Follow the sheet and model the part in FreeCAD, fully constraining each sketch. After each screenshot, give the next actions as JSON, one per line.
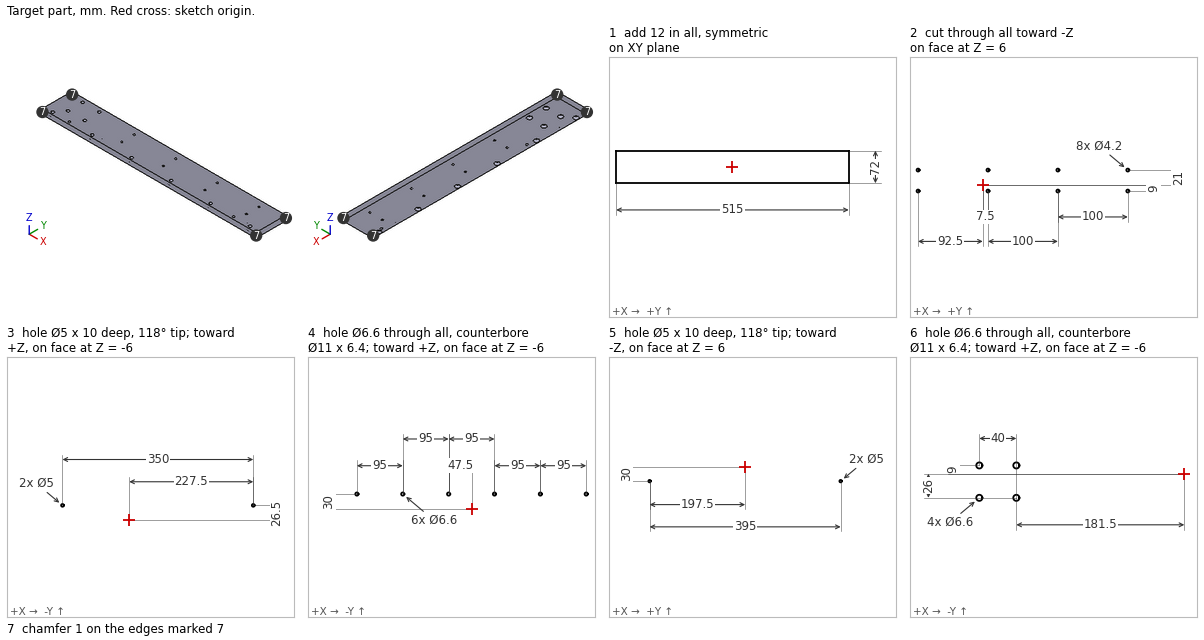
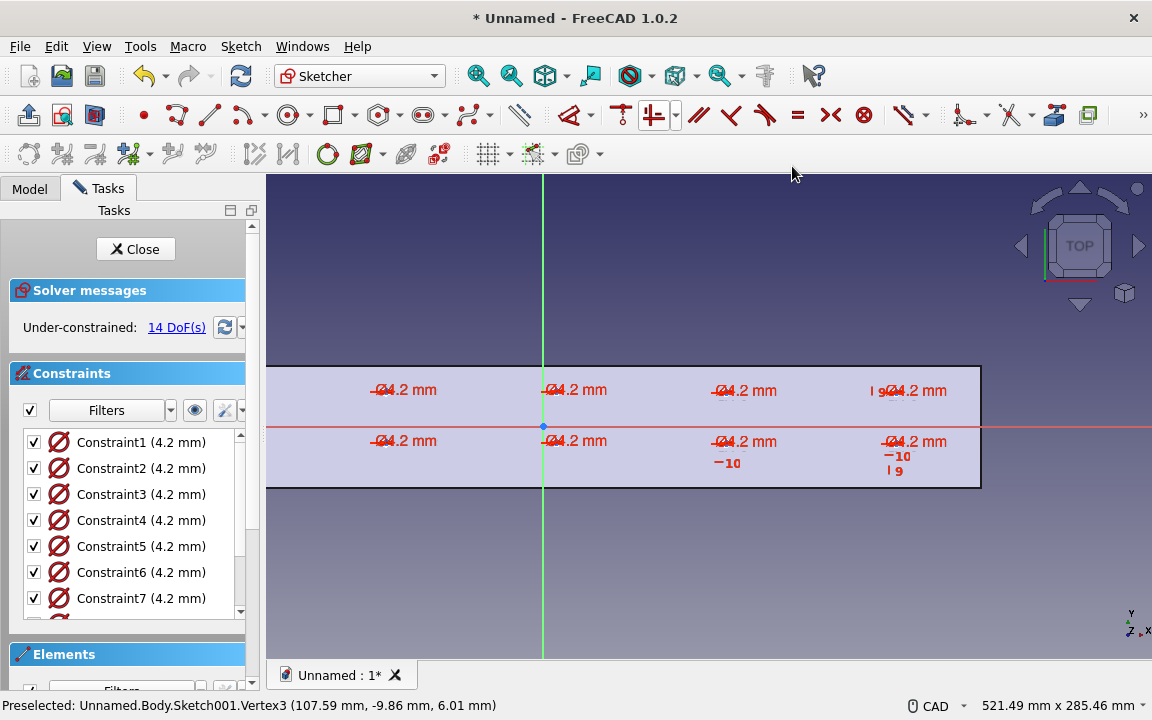
{"action": "left_click", "coordinate": [726, 444]}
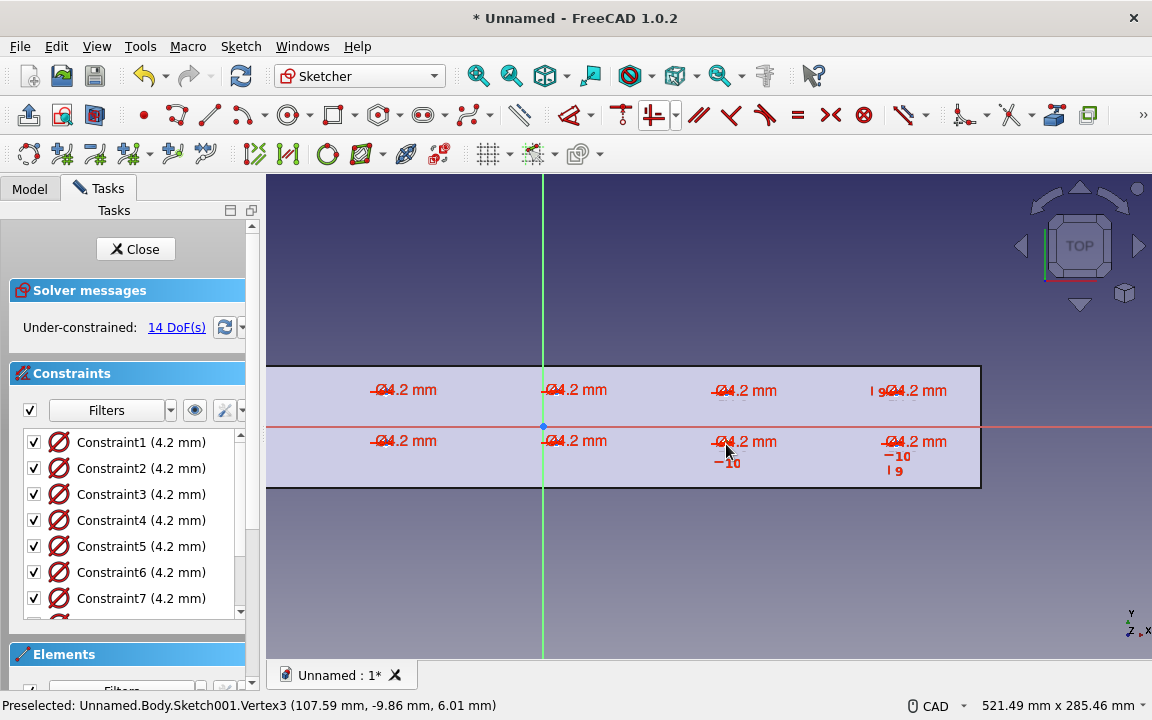
{"action": "left_click", "coordinate": [726, 393]}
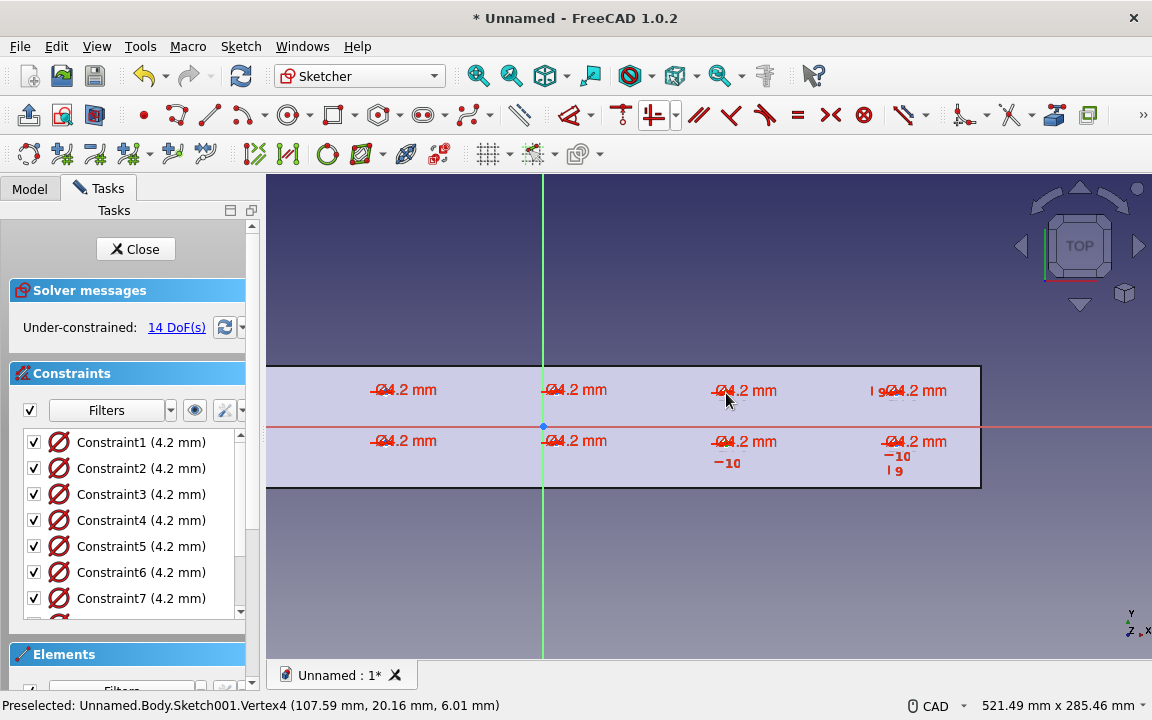
{"action": "key", "text": "v"}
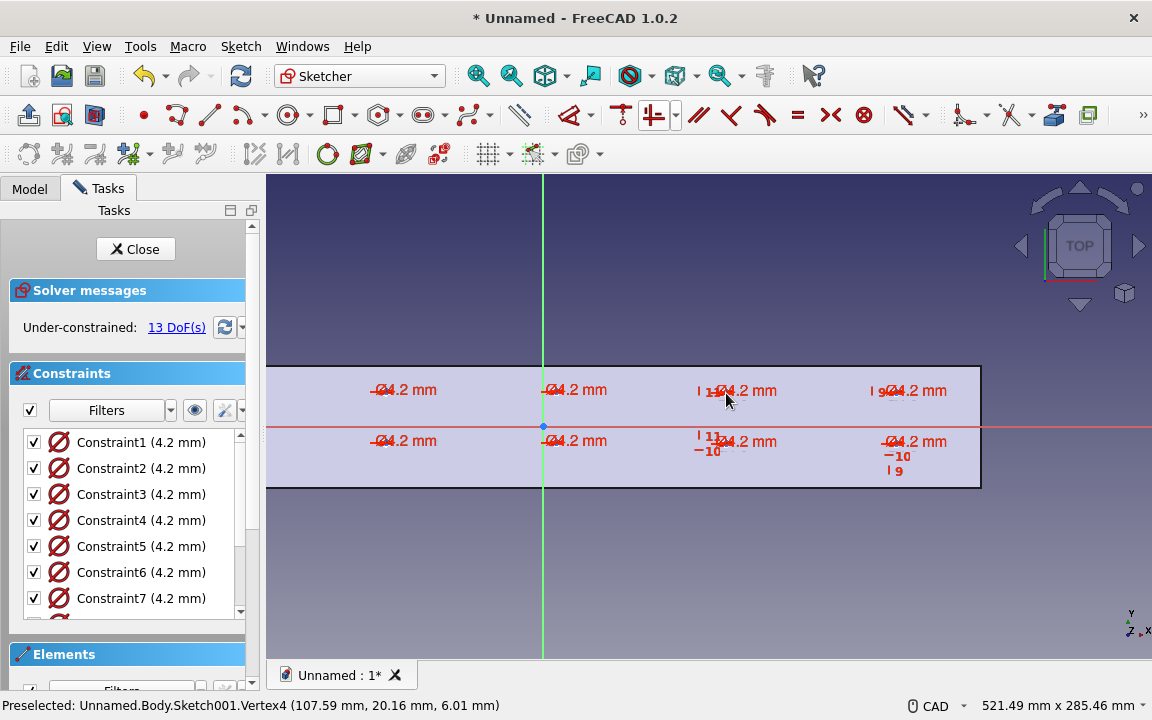
{"action": "left_click", "coordinate": [896, 393]}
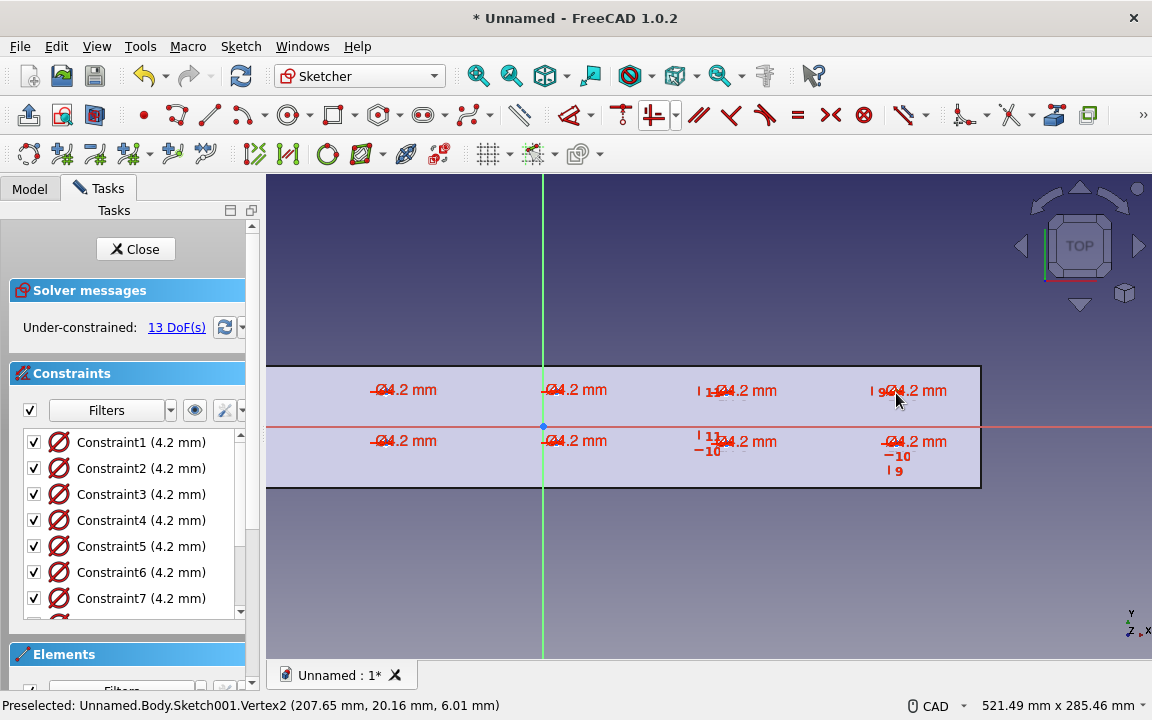
{"action": "left_click", "coordinate": [726, 393]}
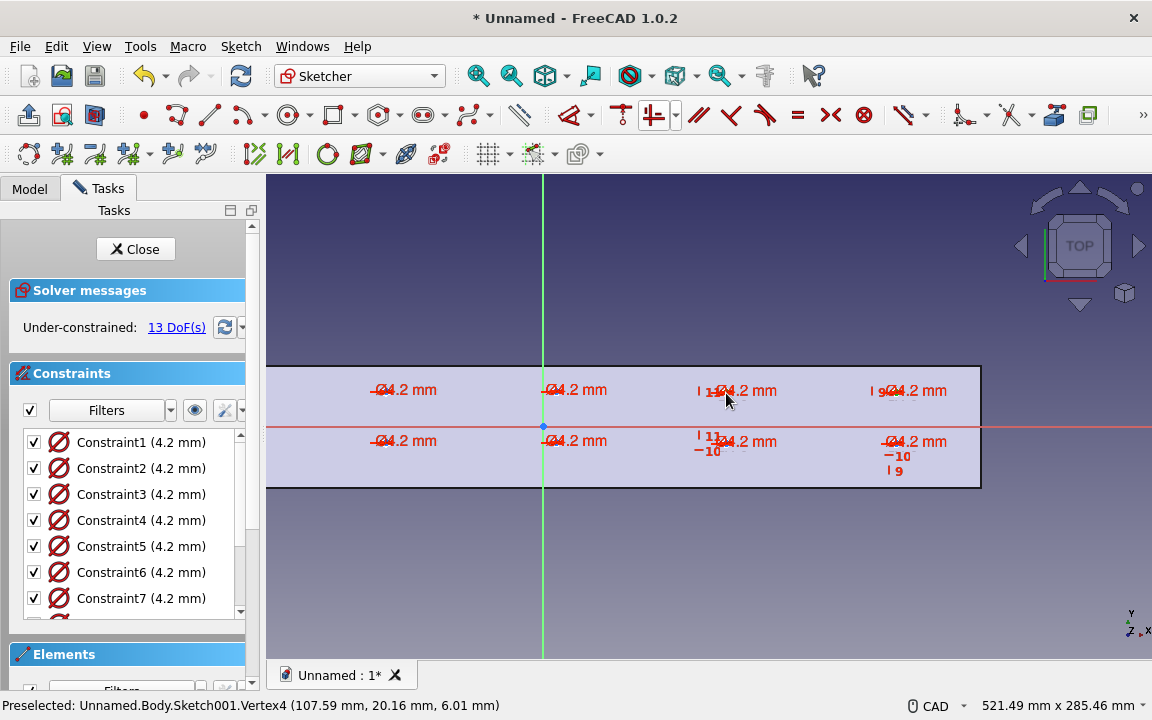
{"action": "left_click", "coordinate": [676, 116]}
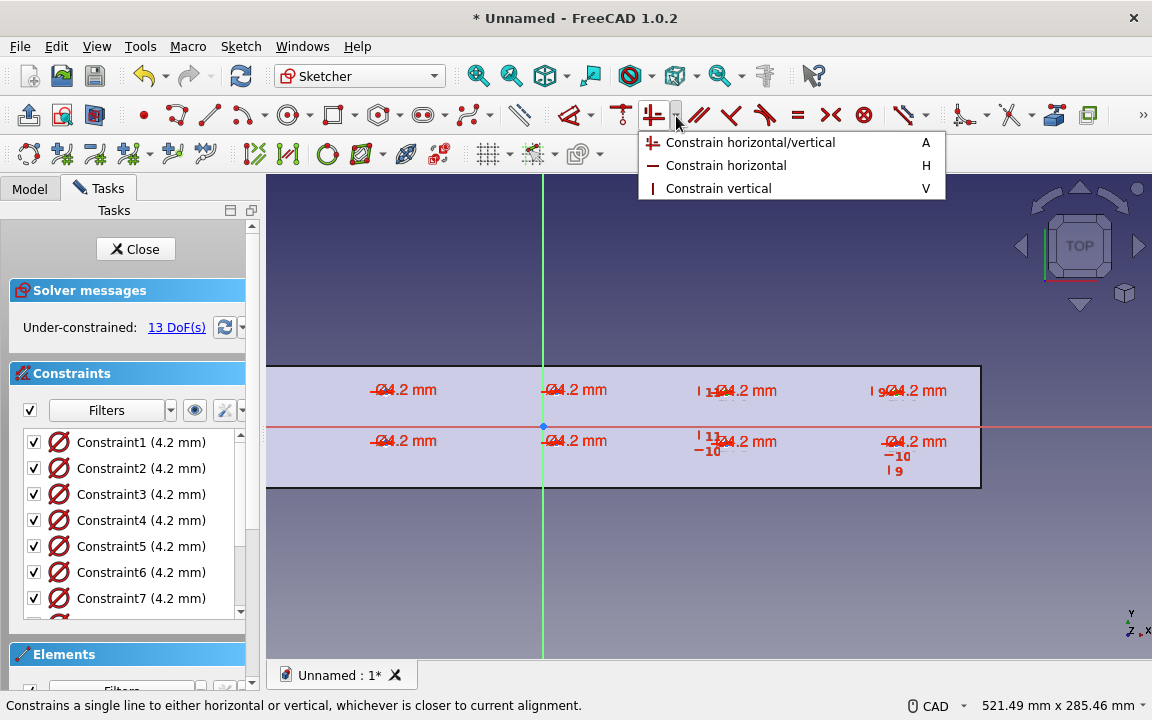
{"action": "left_click", "coordinate": [792, 166]}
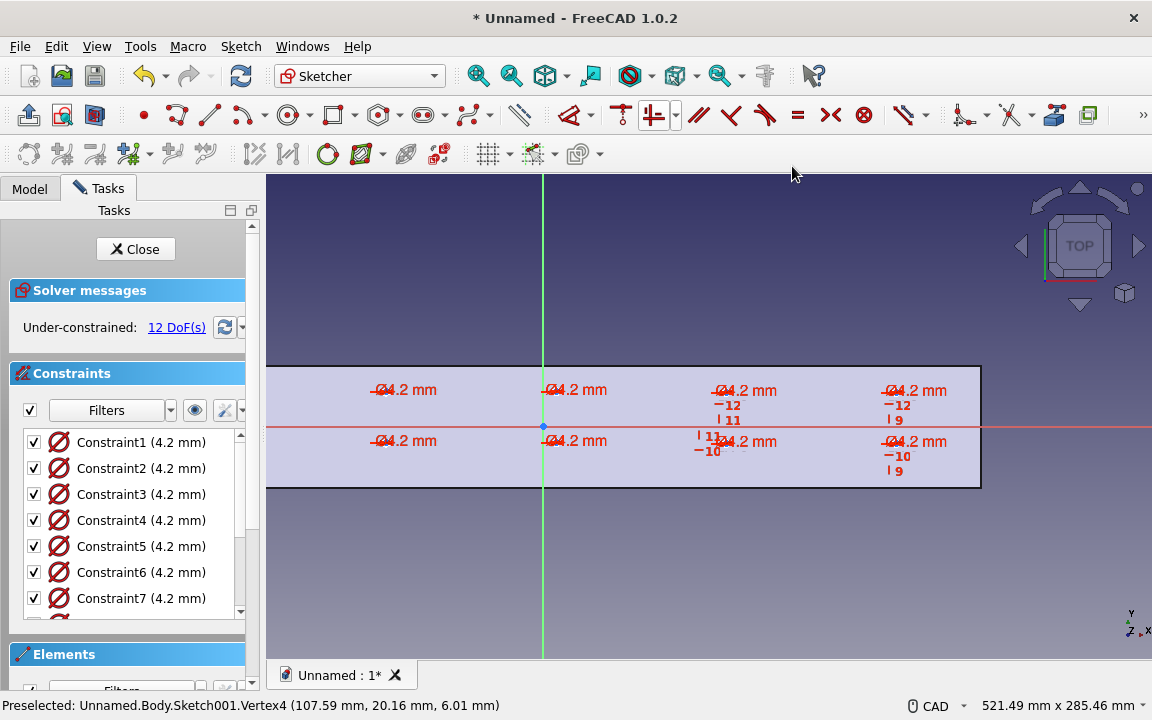
{"action": "left_click", "coordinate": [726, 444]}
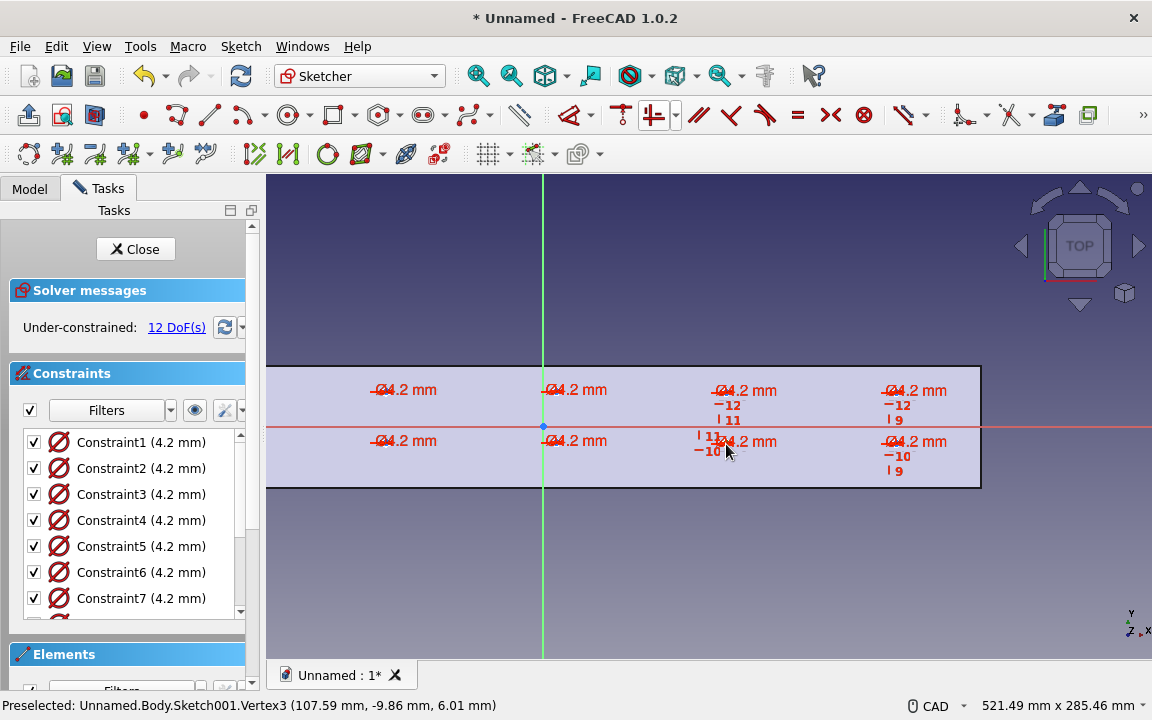
{"action": "left_click", "coordinate": [556, 443]}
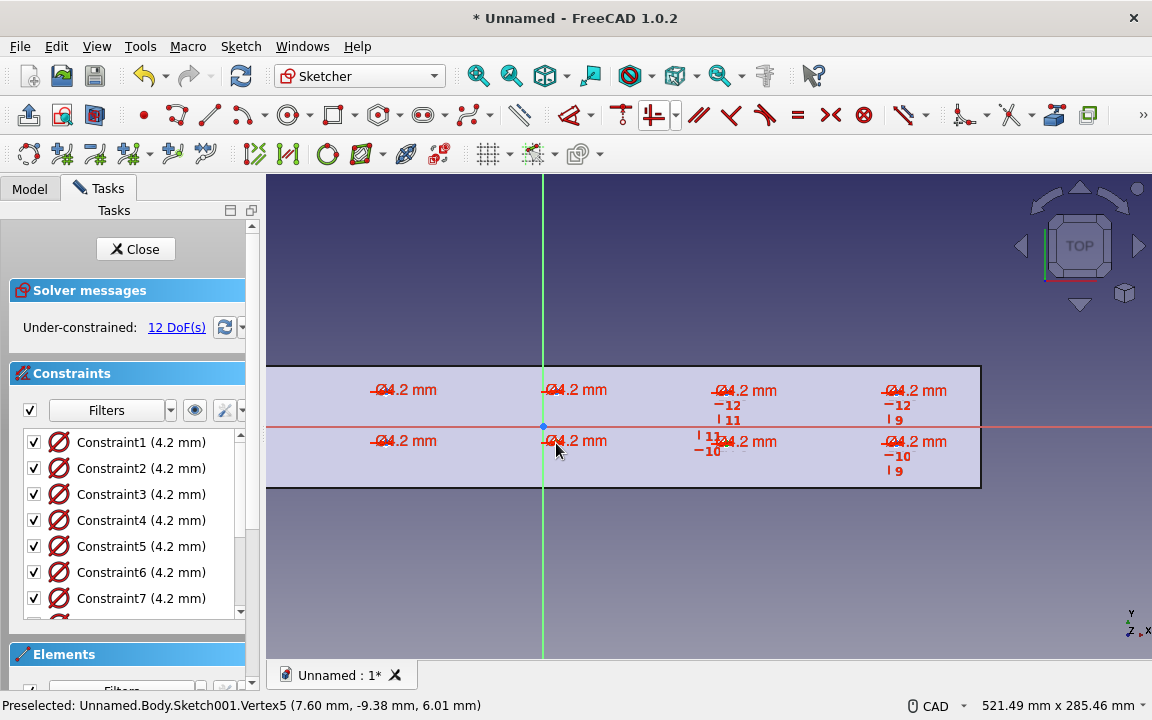
{"action": "left_click", "coordinate": [676, 116]}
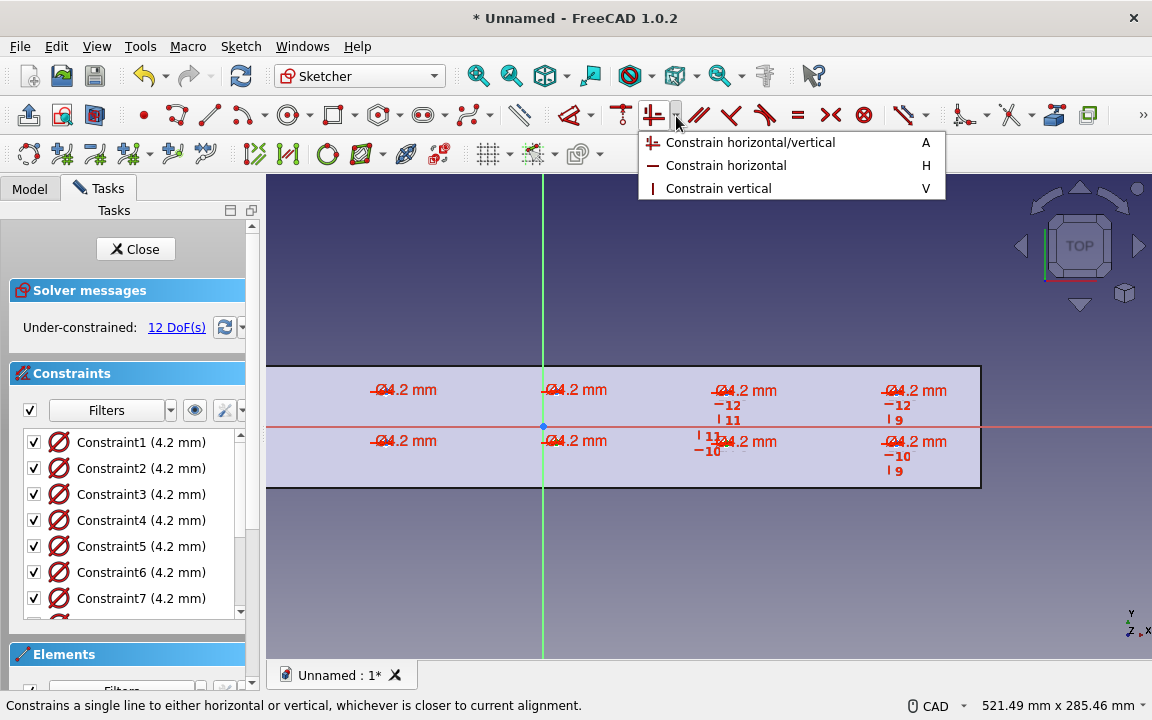
{"action": "left_click", "coordinate": [792, 166]}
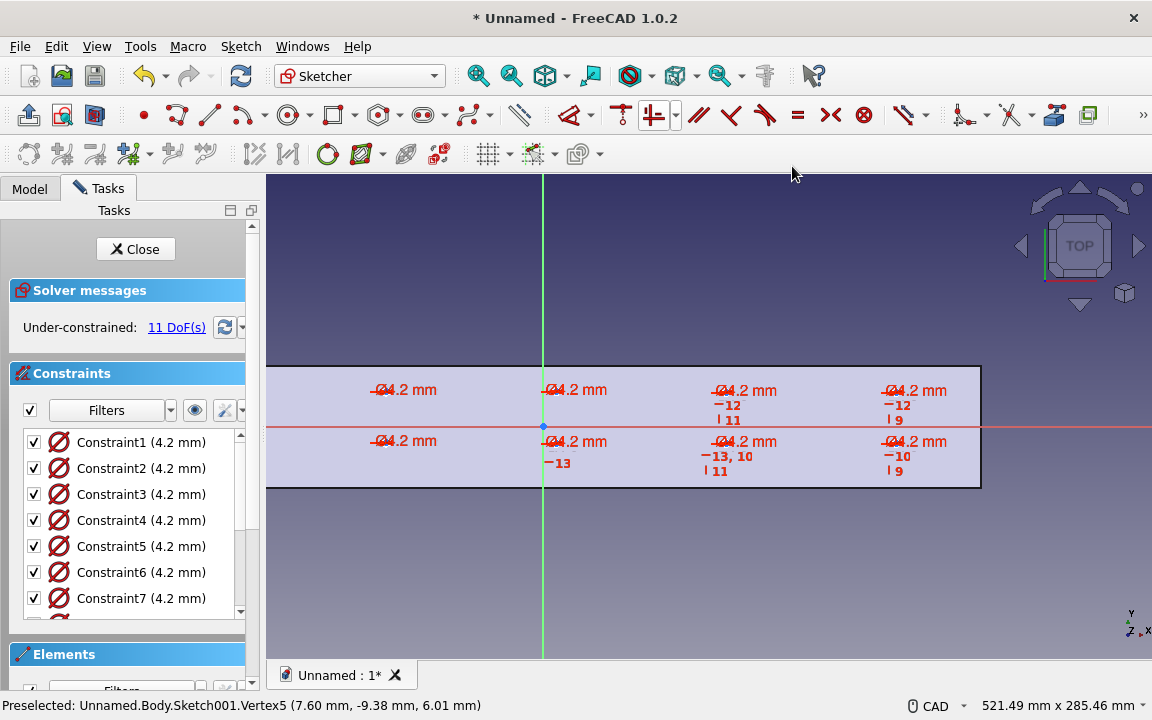
{"action": "left_click", "coordinate": [556, 444]}